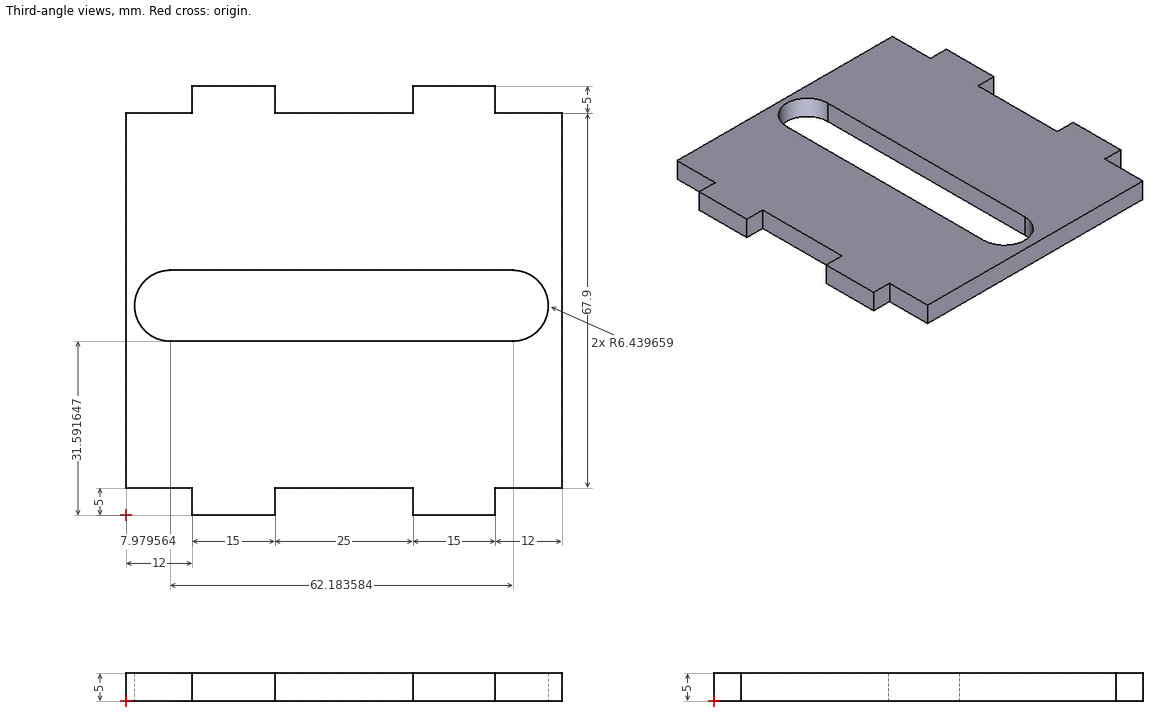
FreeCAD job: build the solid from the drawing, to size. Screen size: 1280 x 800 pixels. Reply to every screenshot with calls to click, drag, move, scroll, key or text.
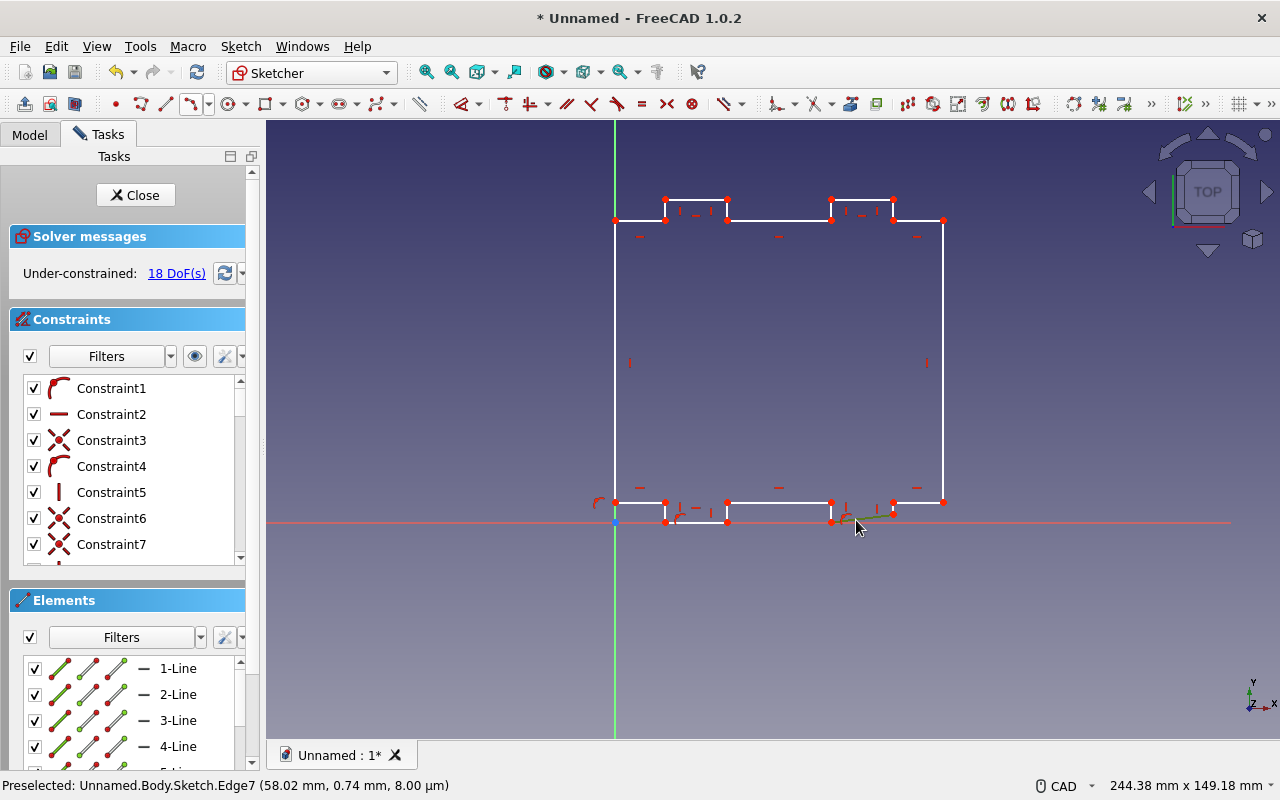
key(h)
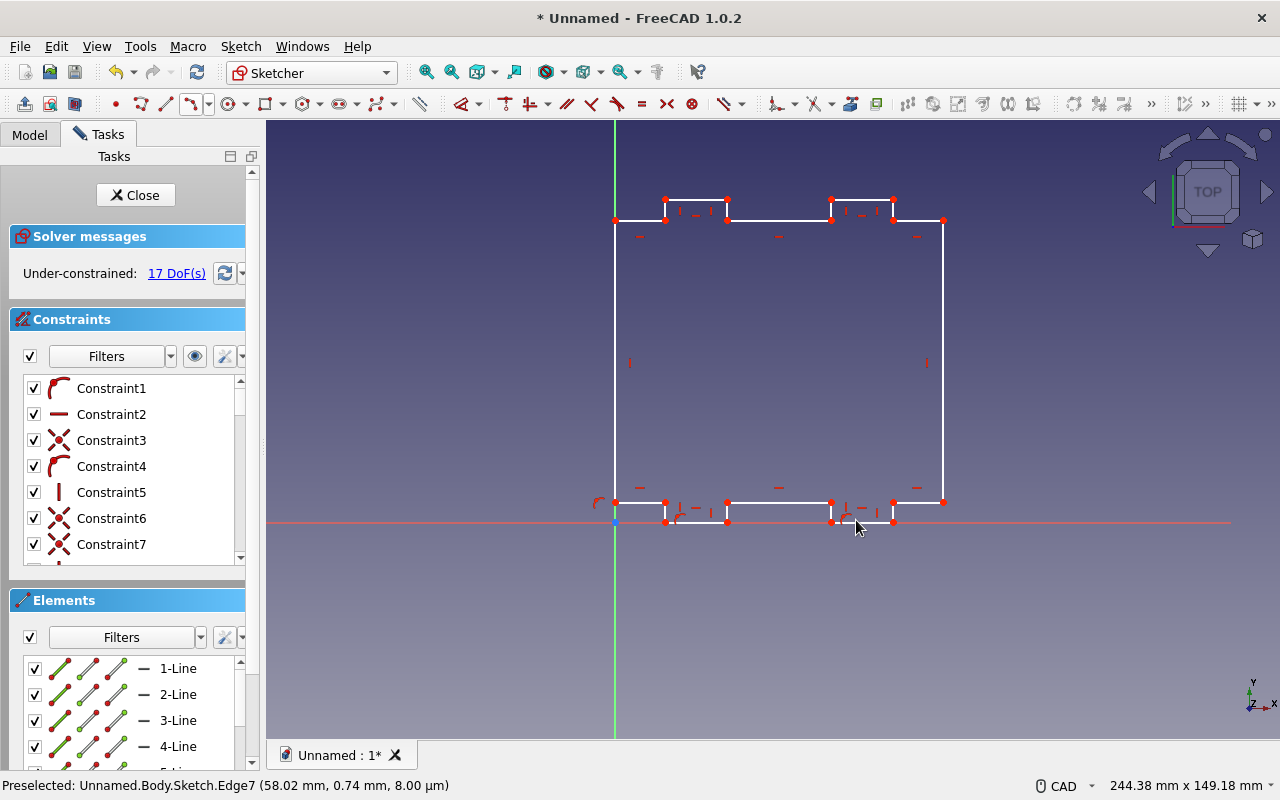
click(460, 104)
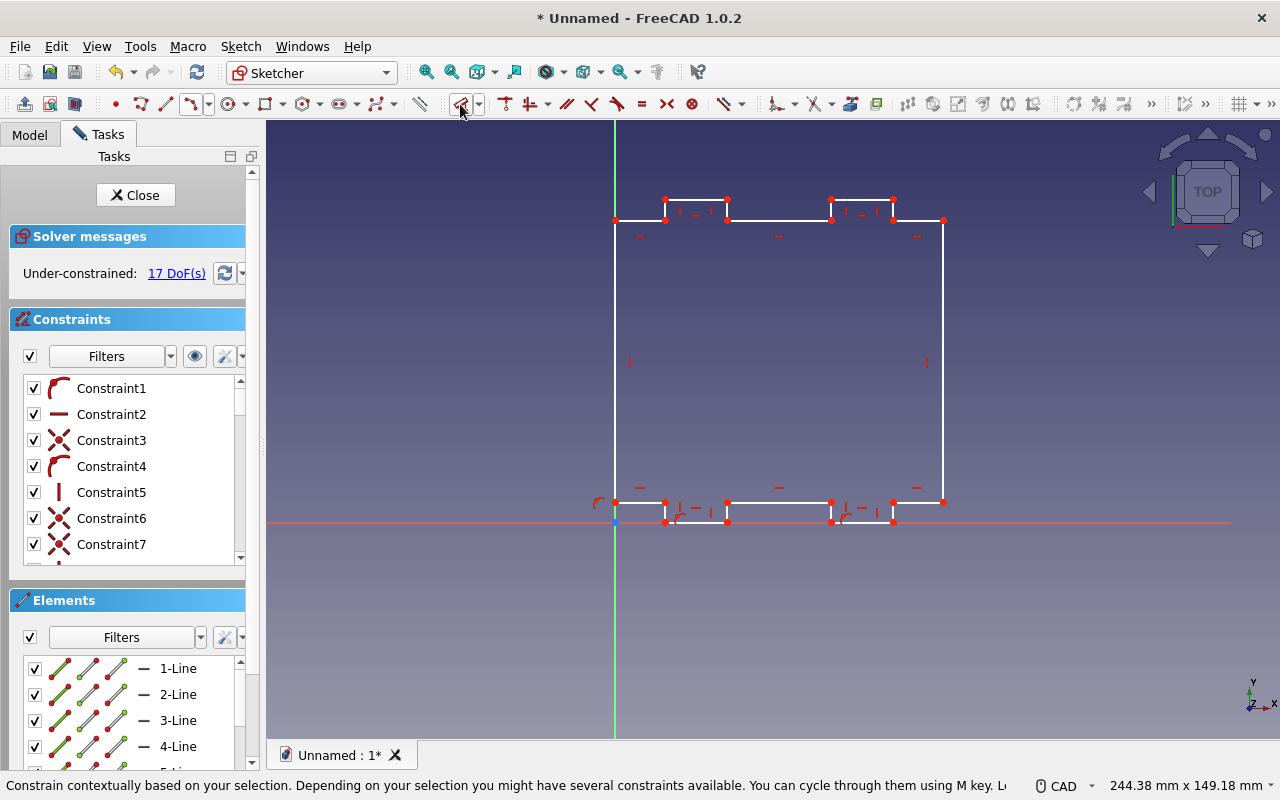
scroll(665, 513, up, 4)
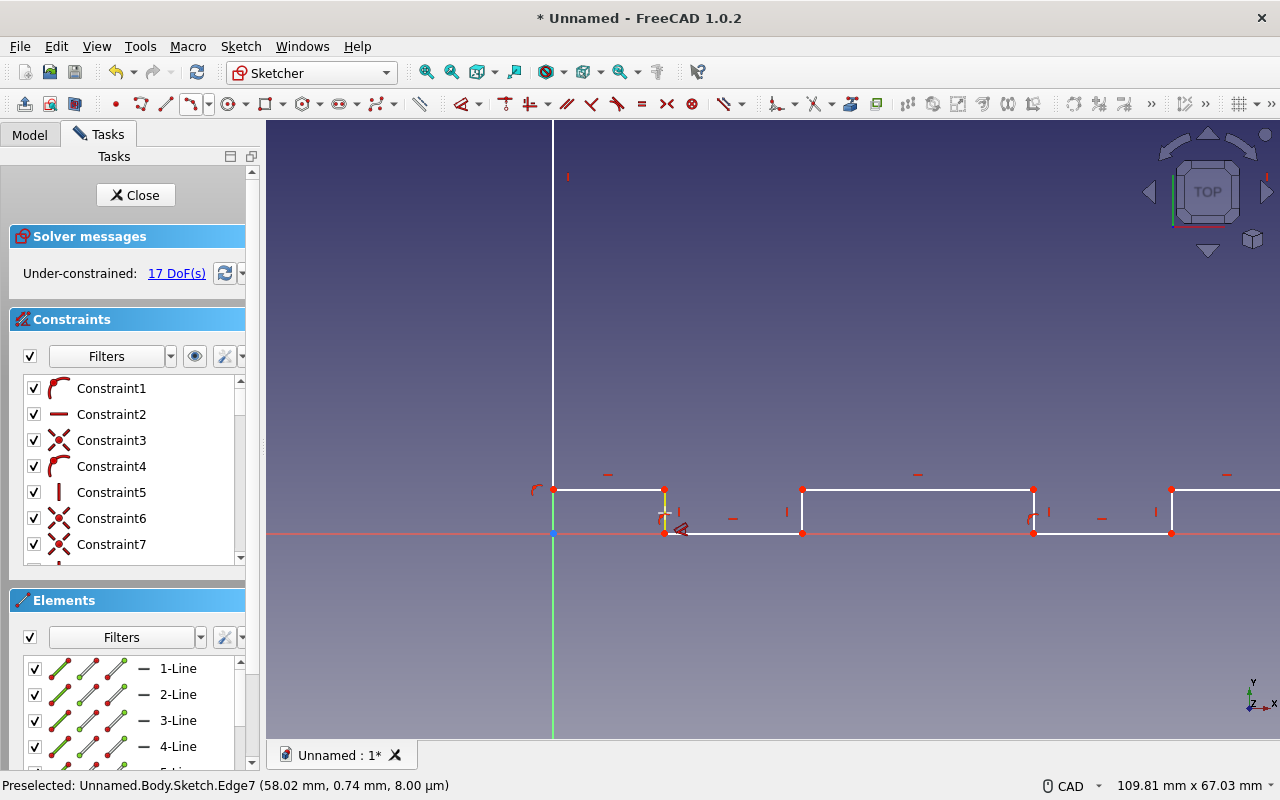
click(665, 512)
click(631, 512)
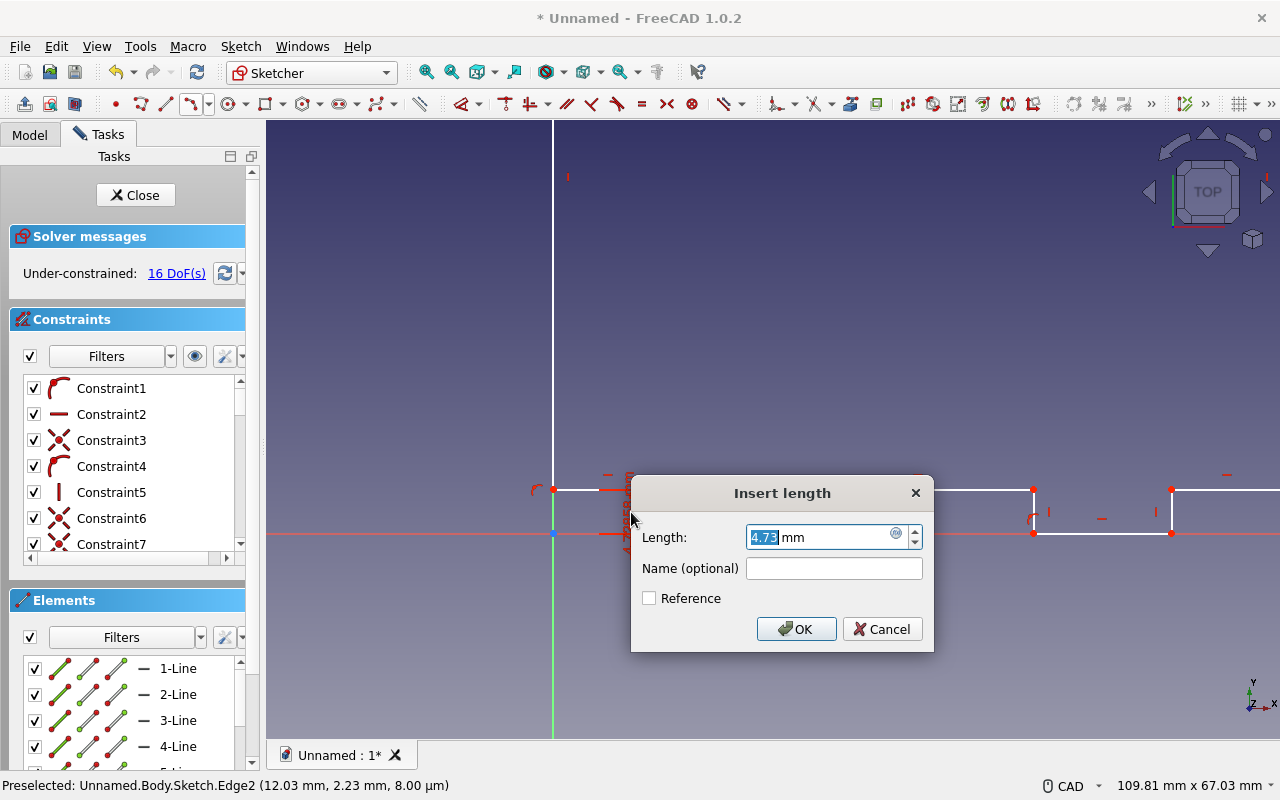
text(5)
key(Return)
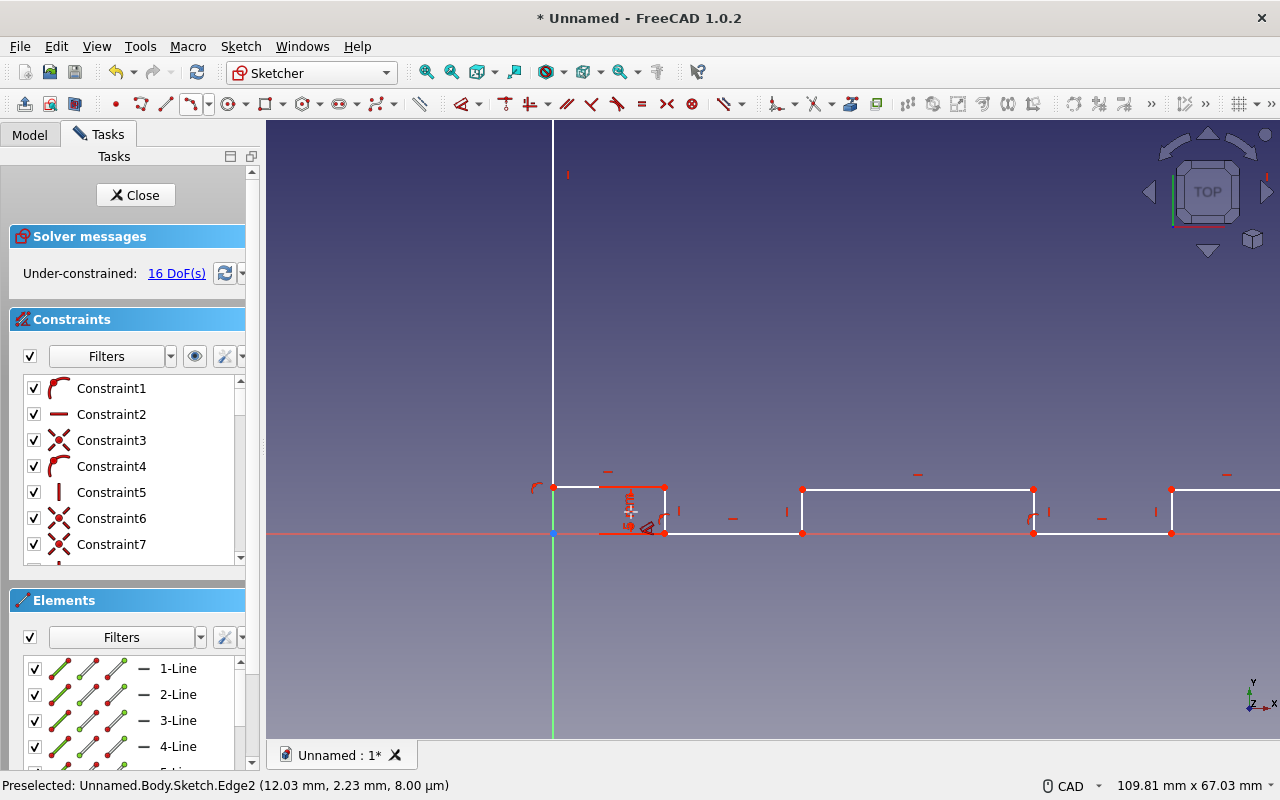
click(803, 521)
click(769, 512)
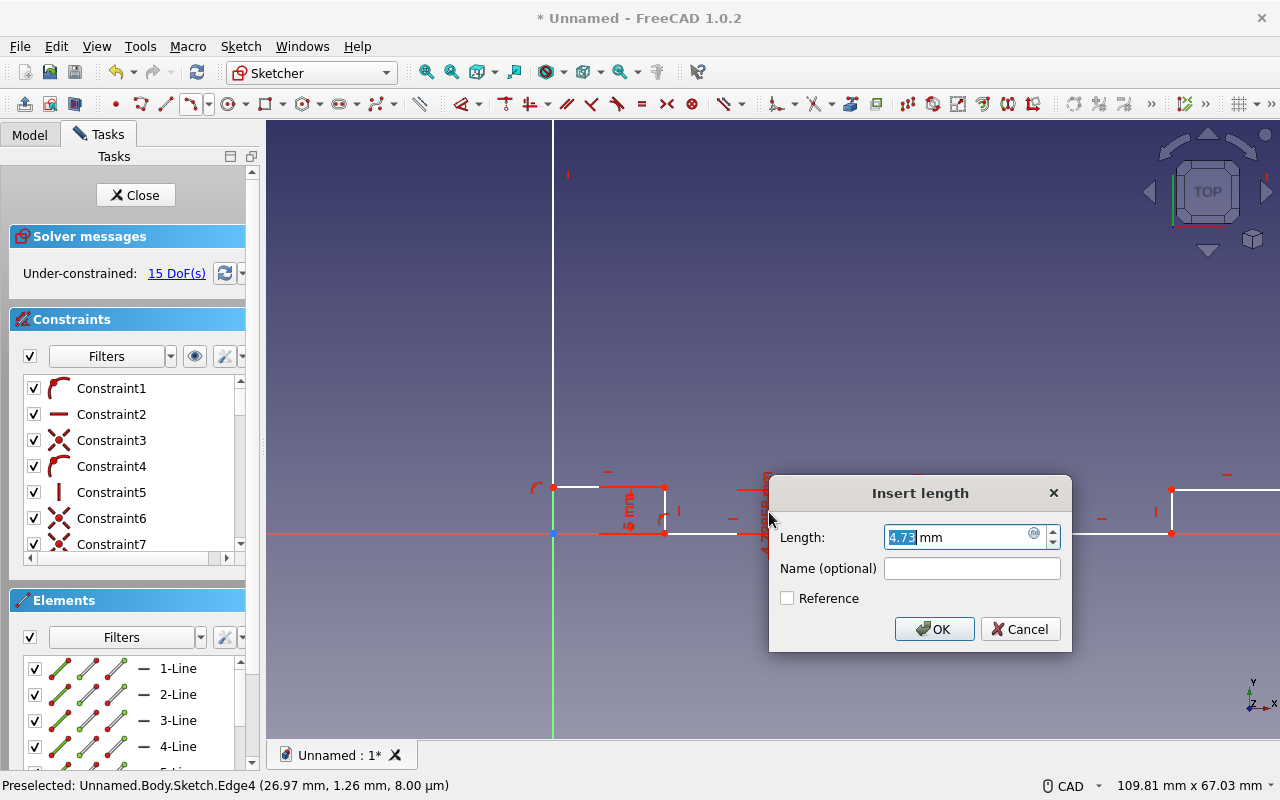
text(5)
key(Return)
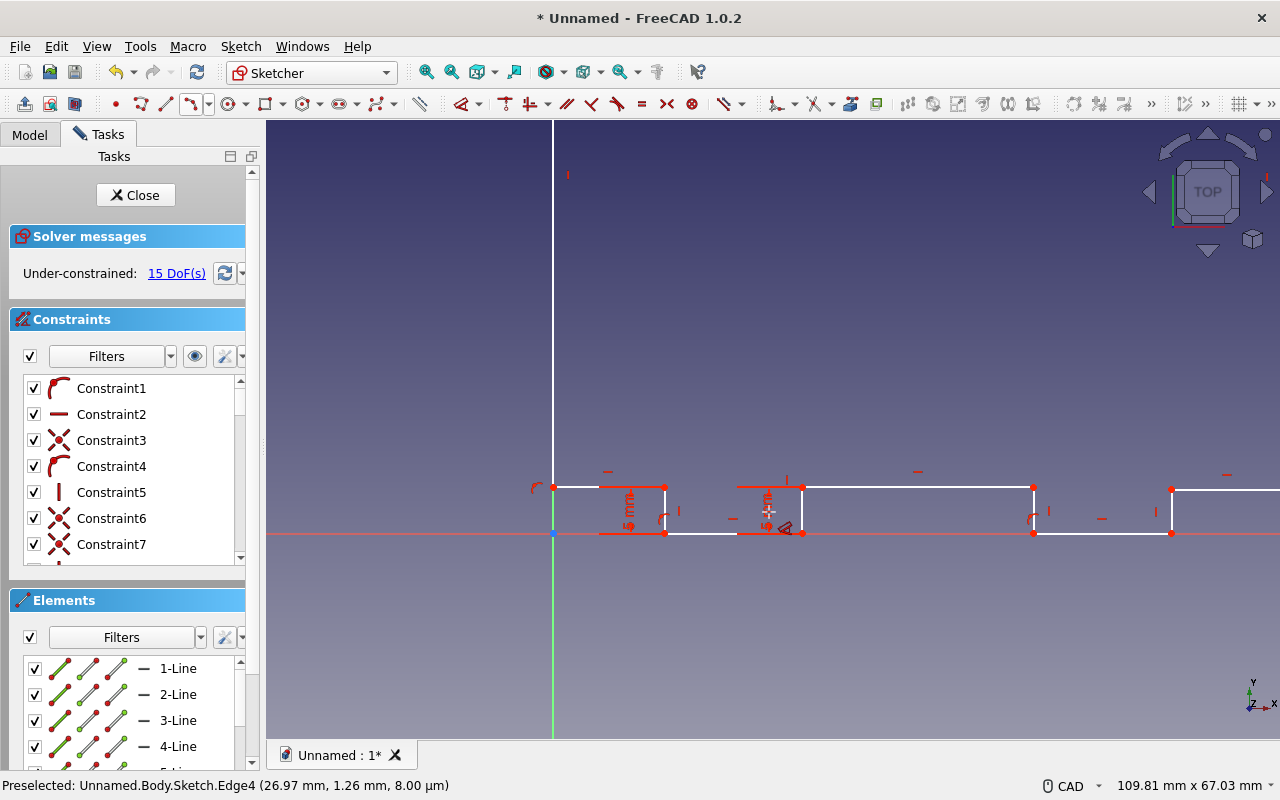
scroll(445, 711, down, 3)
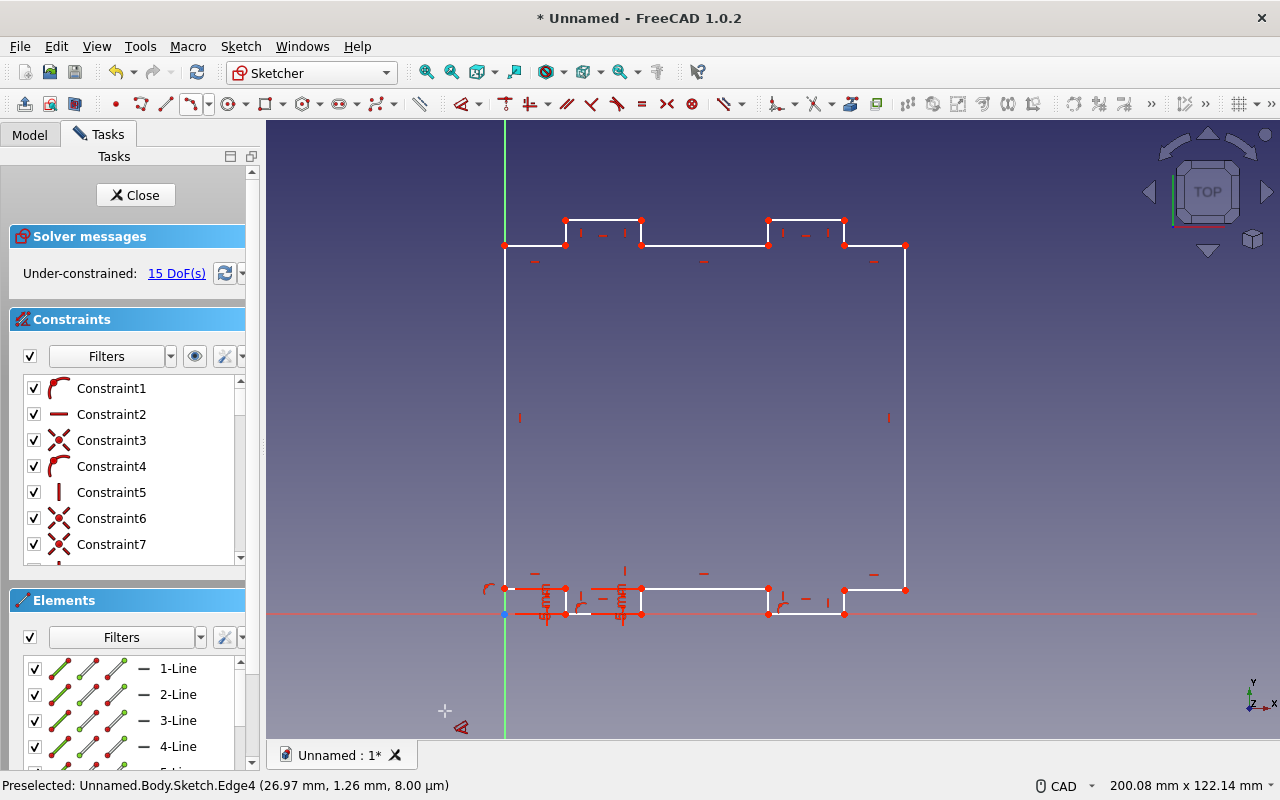
scroll(844, 607, up, 4)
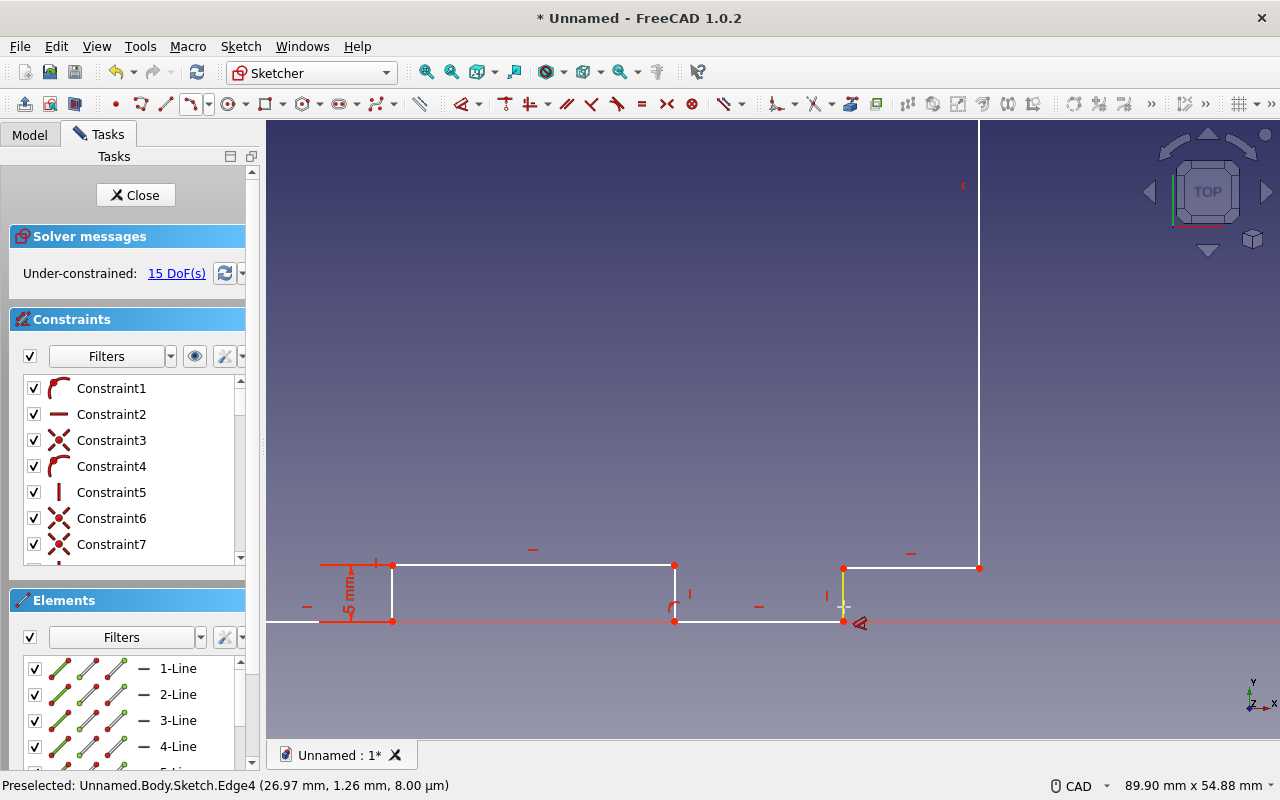
click(843, 606)
click(877, 595)